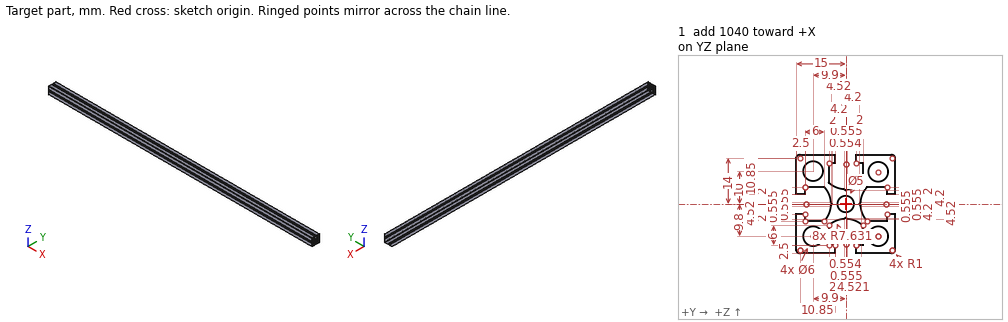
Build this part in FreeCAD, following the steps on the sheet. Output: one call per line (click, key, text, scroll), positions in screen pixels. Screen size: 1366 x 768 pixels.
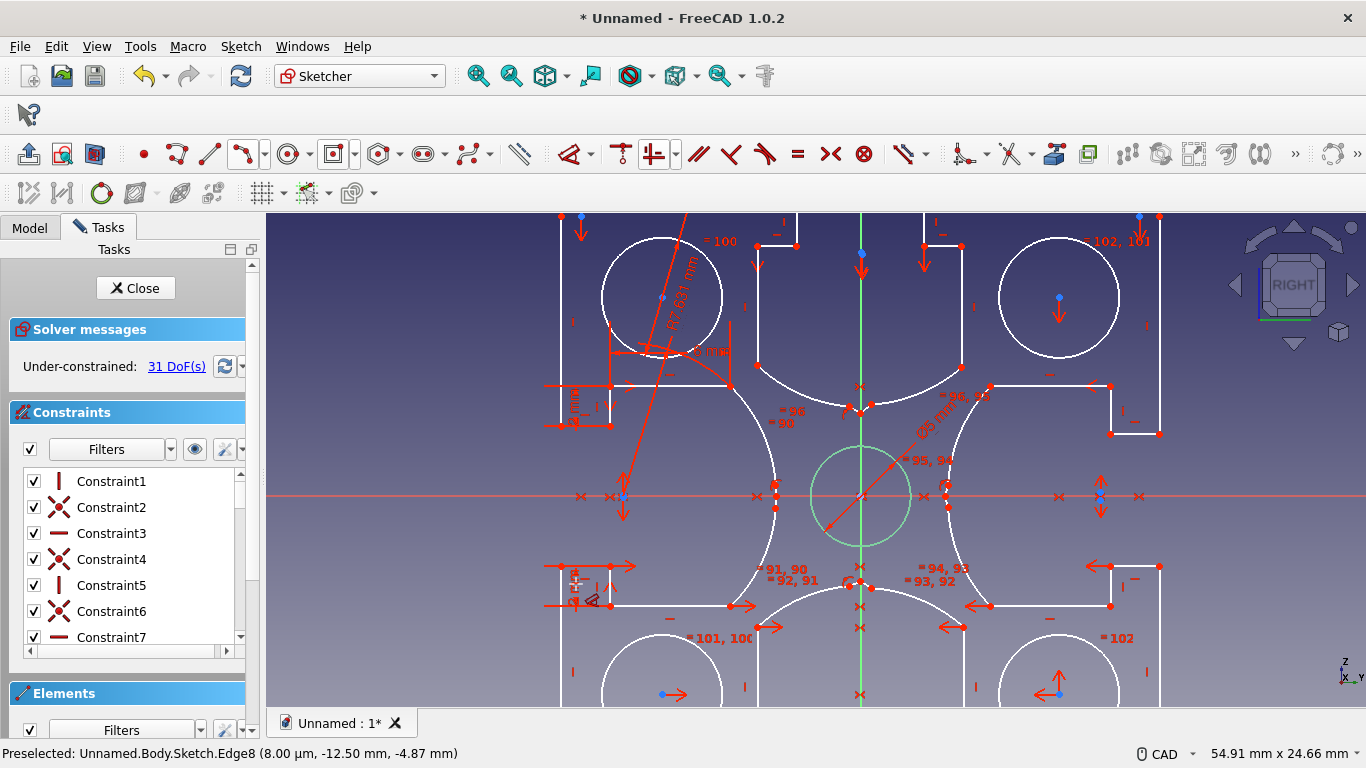
scroll(610, 416, down, 3)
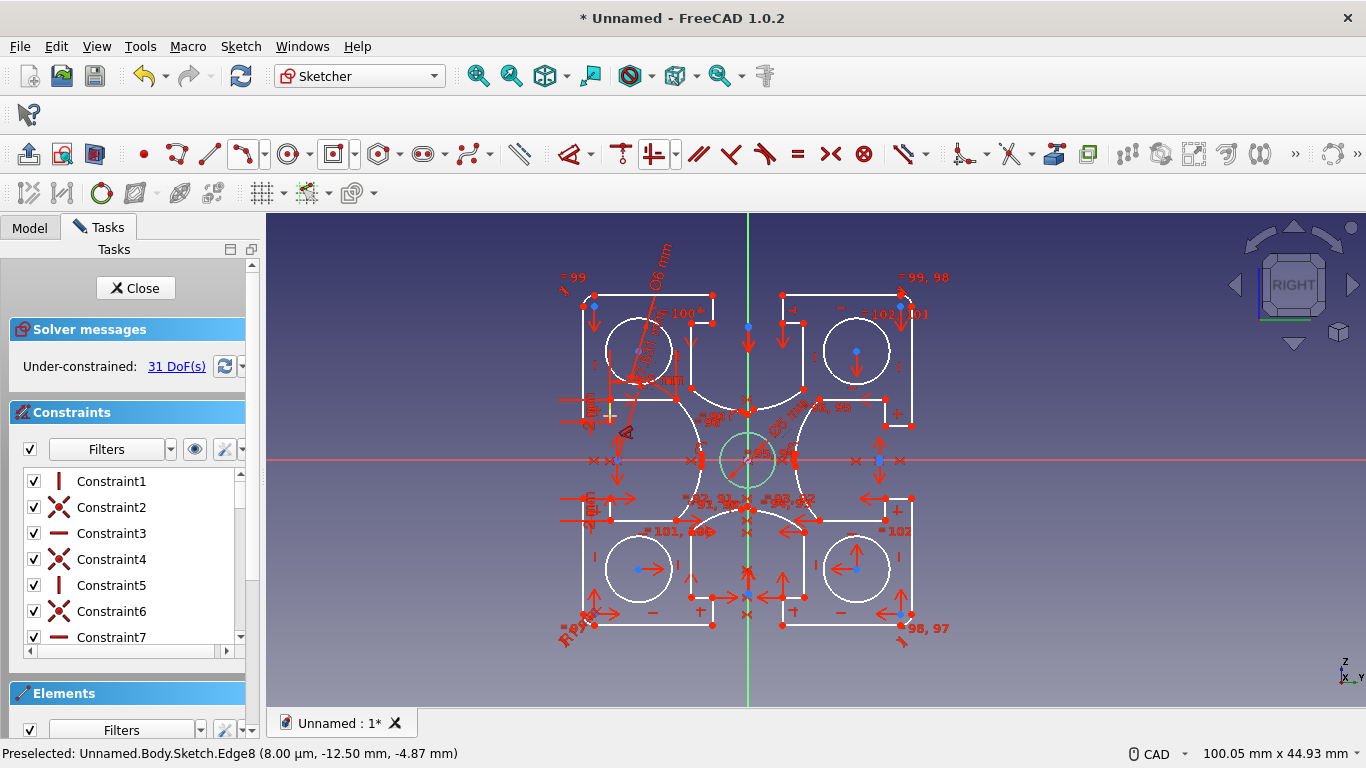
scroll(706, 598, up, 4)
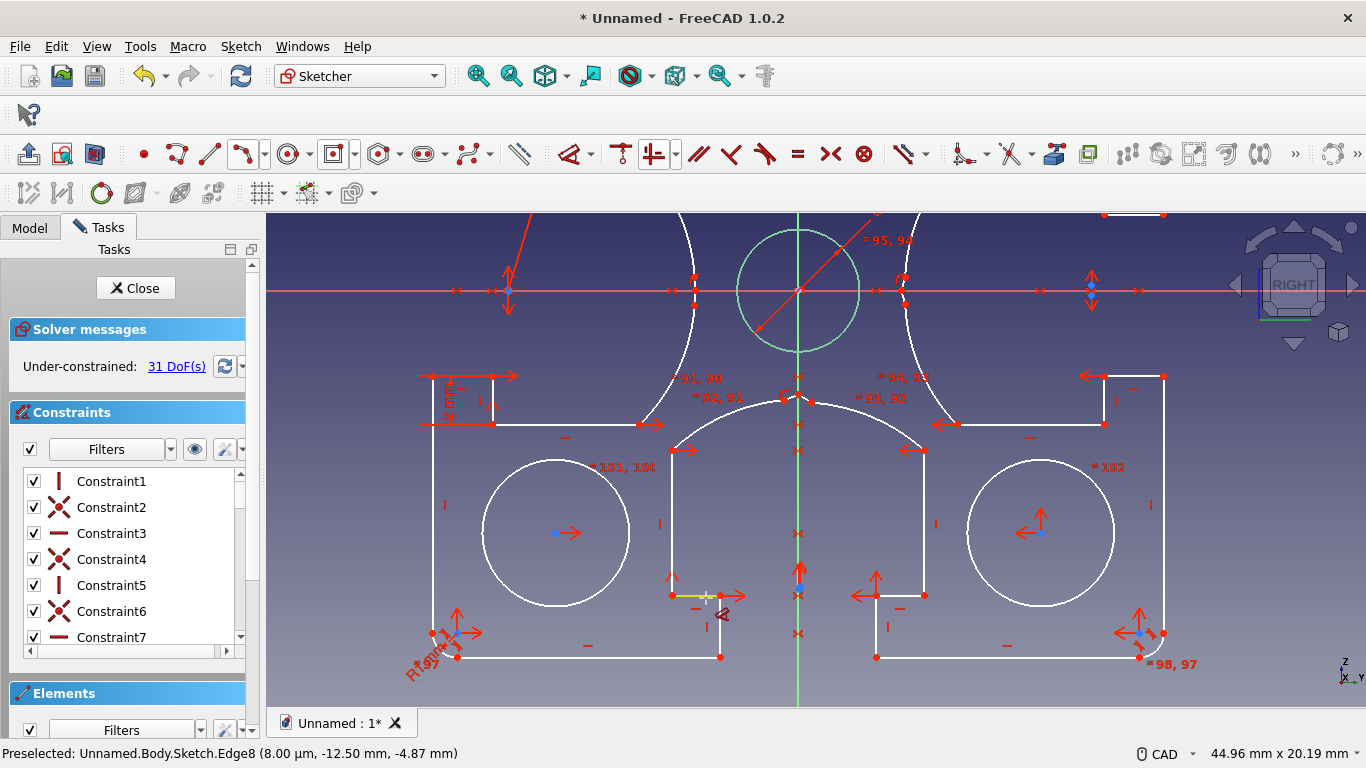
click(706, 596)
click(696, 630)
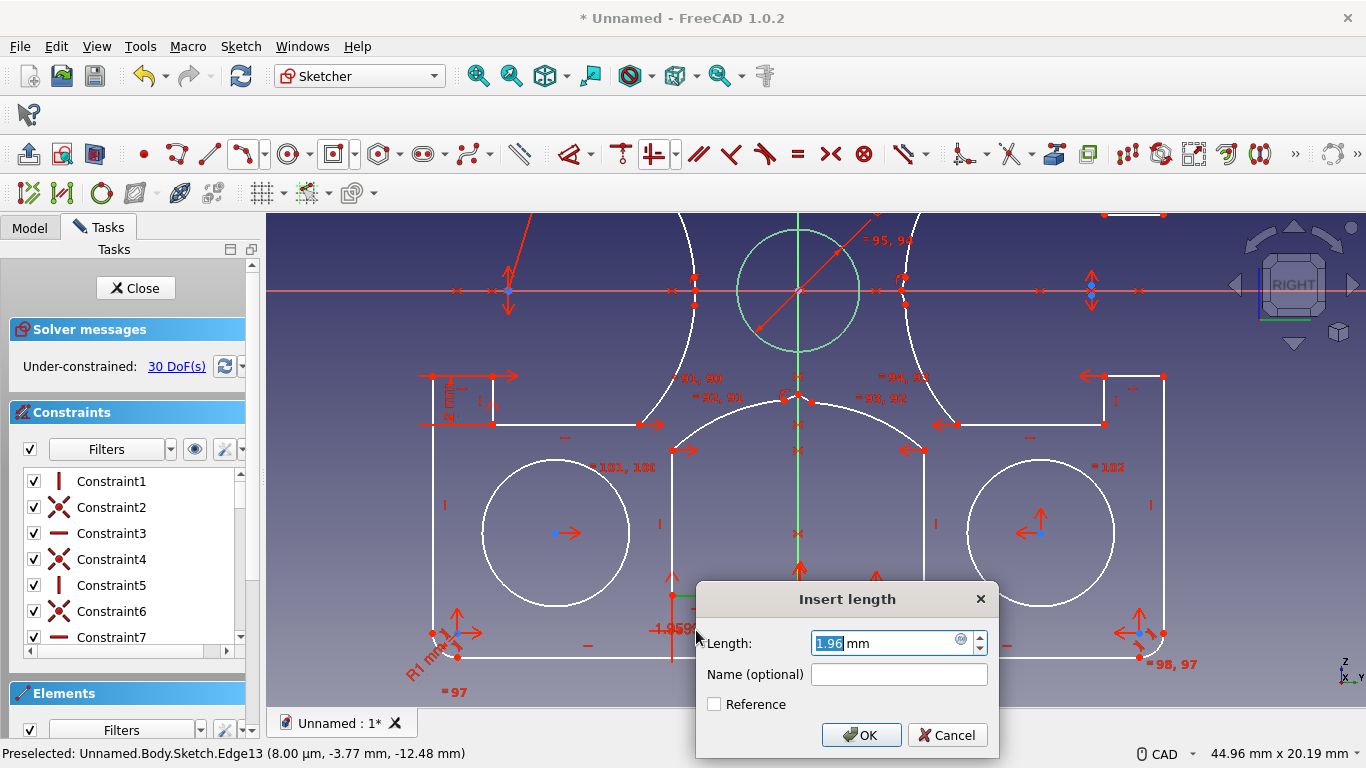
text(2)
key(Return)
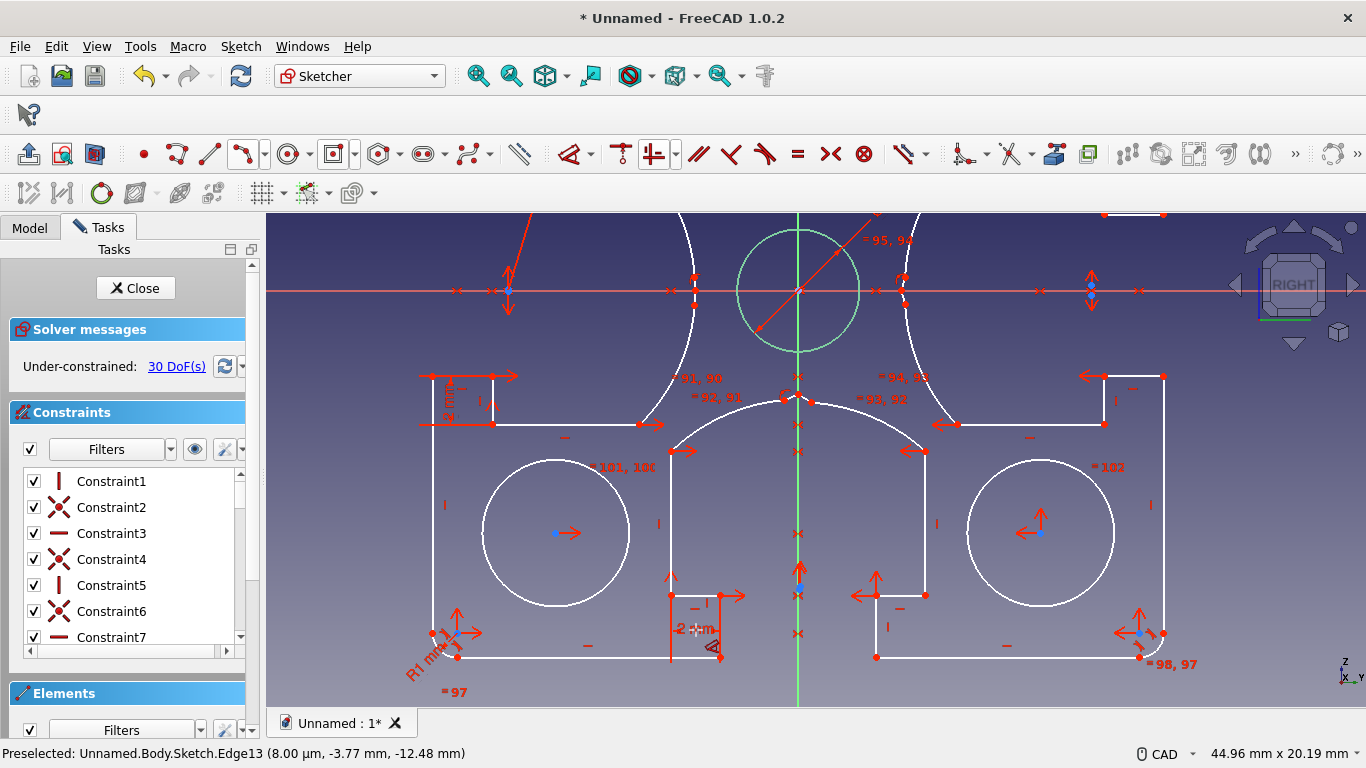
click(671, 553)
click(637, 490)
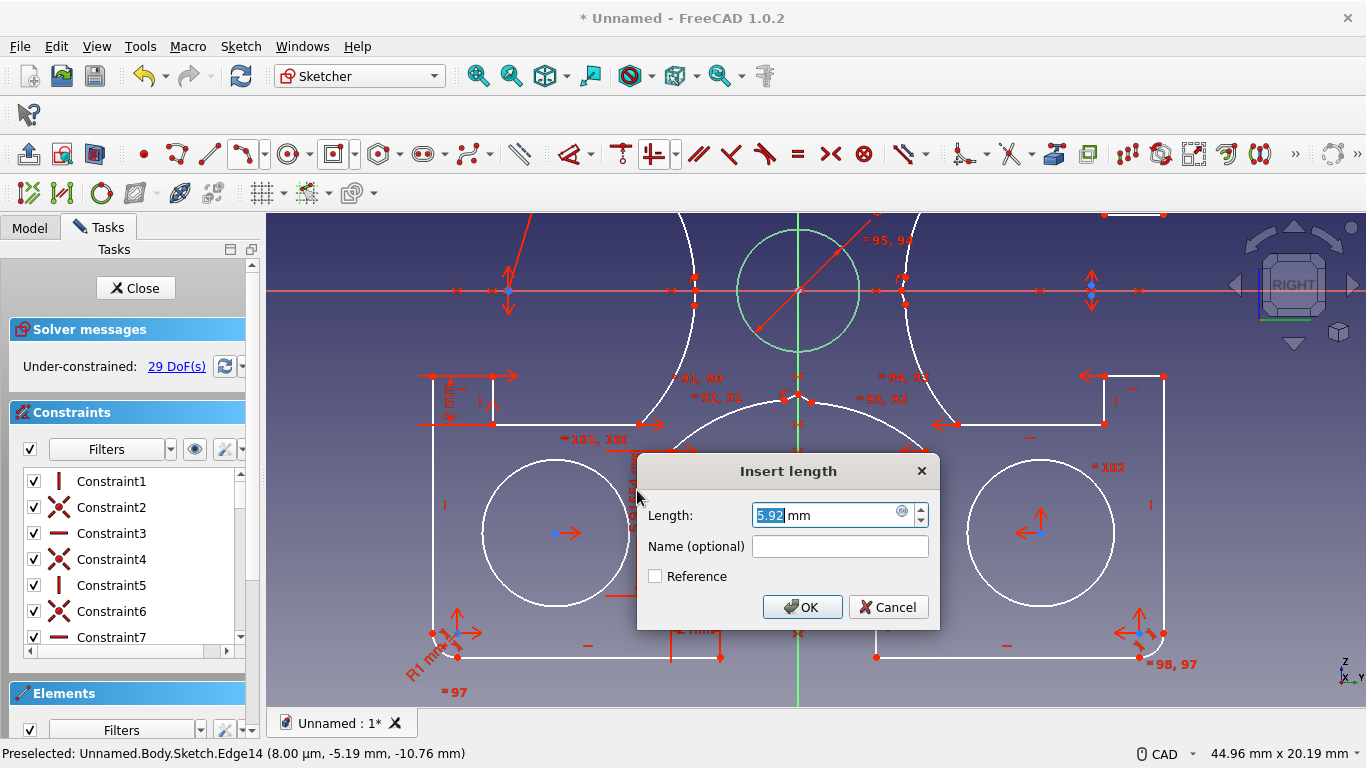
text(6)
key(Return)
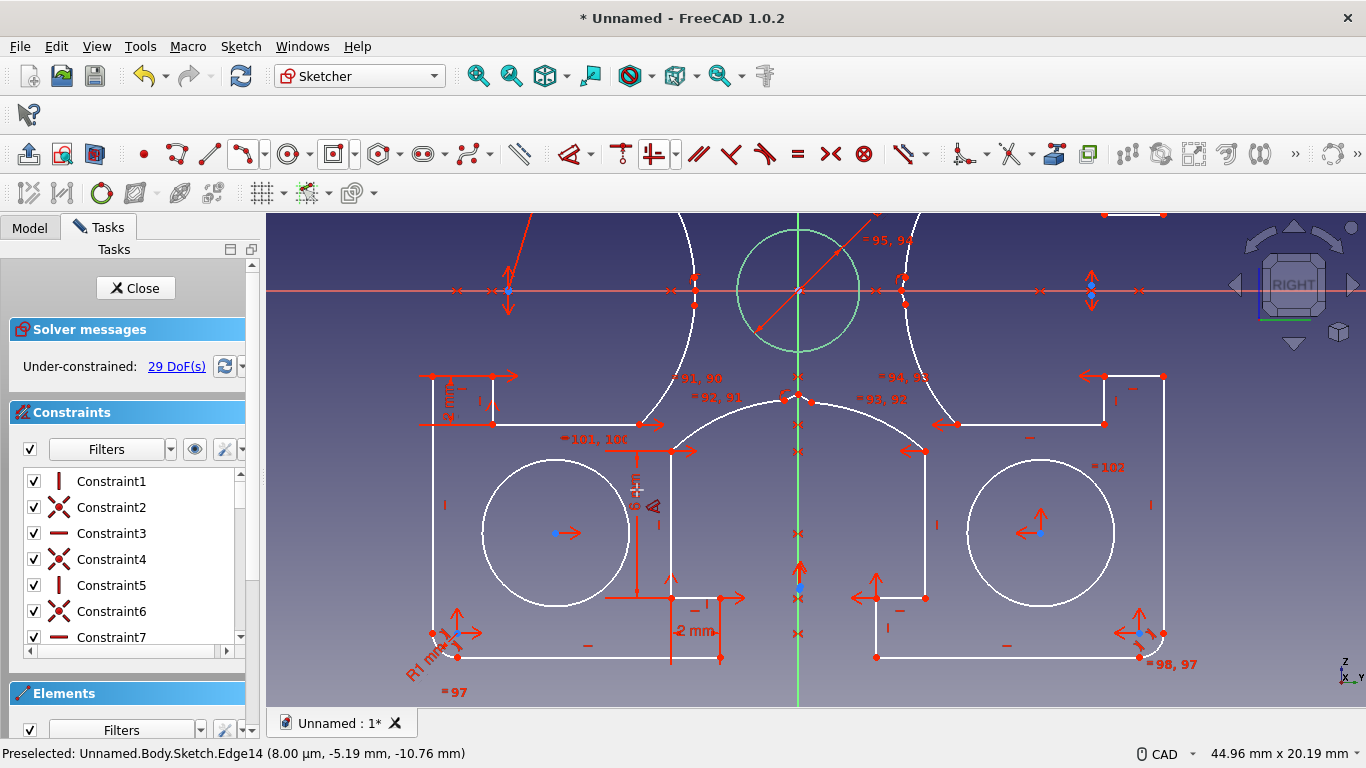
scroll(706, 598, down, 4)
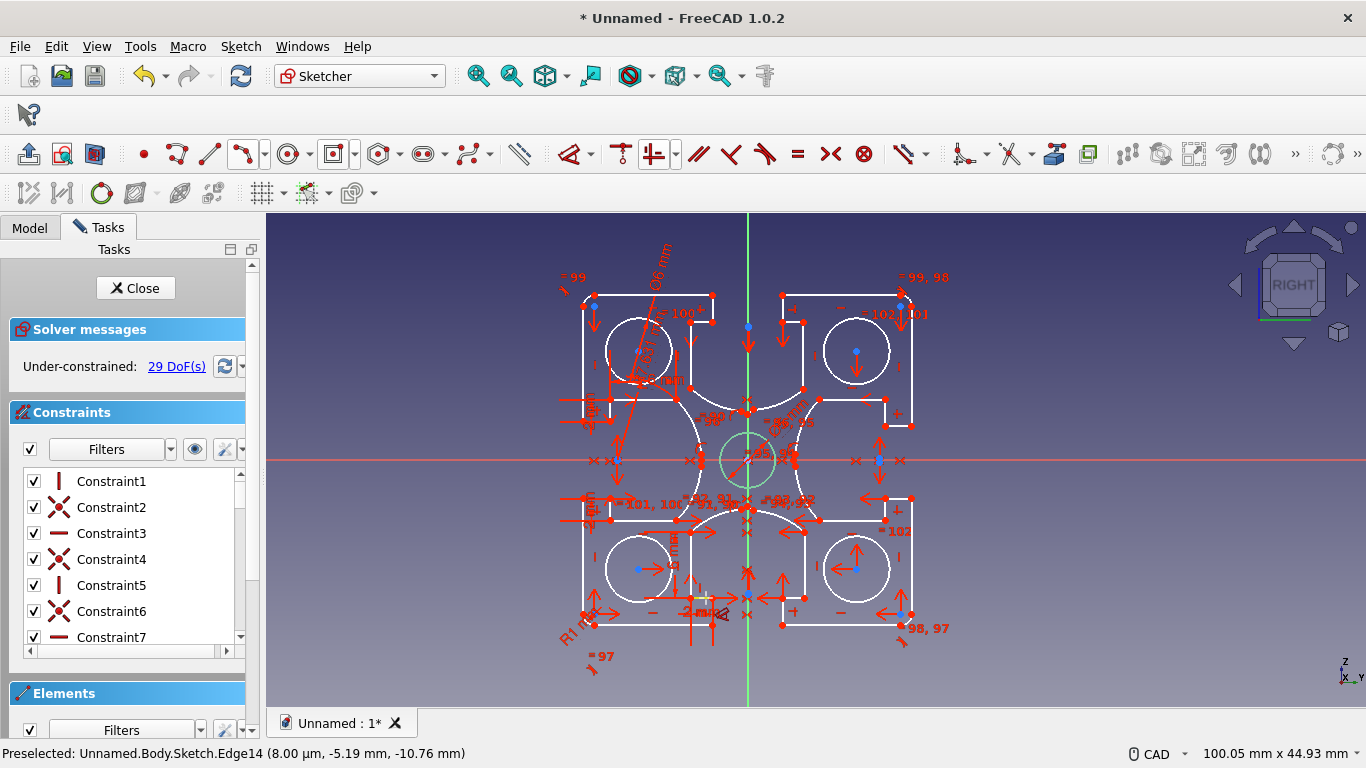
scroll(885, 408, up, 3)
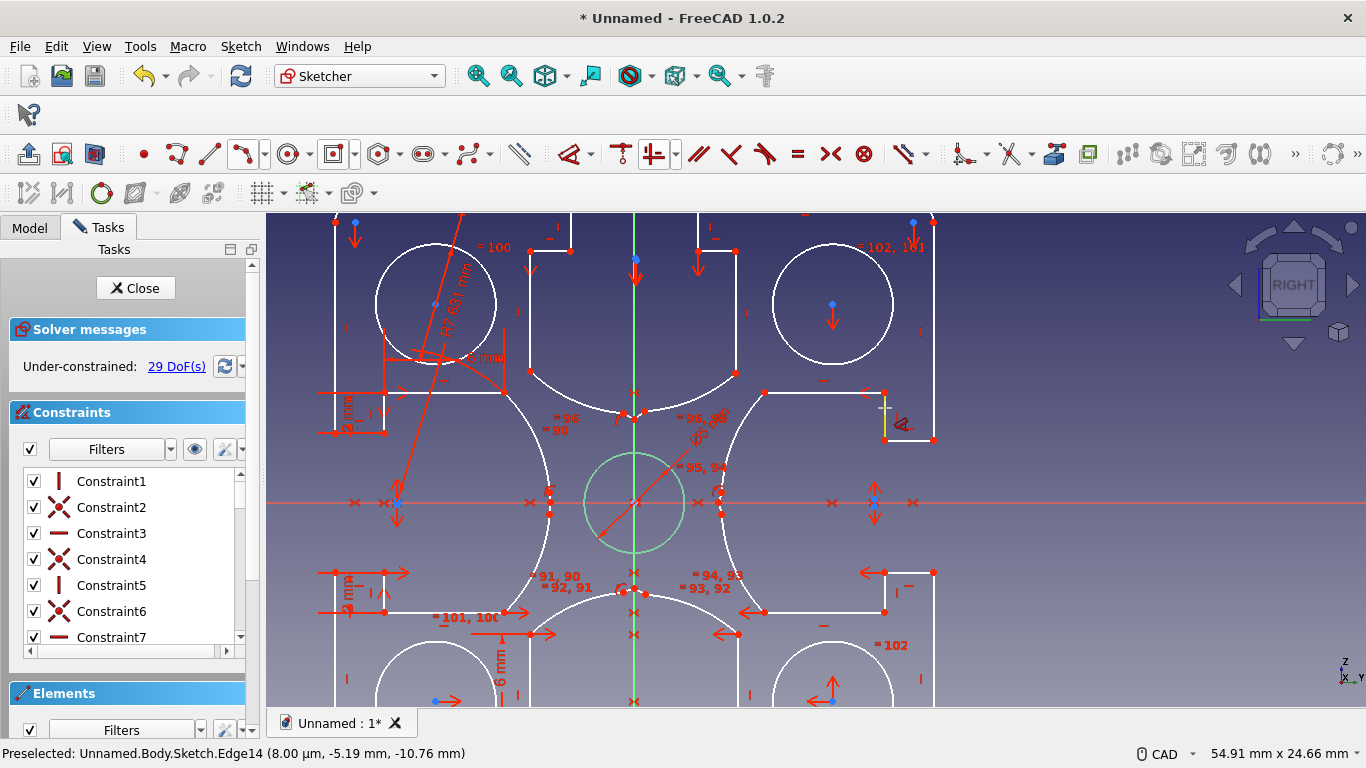
click(885, 407)
click(919, 417)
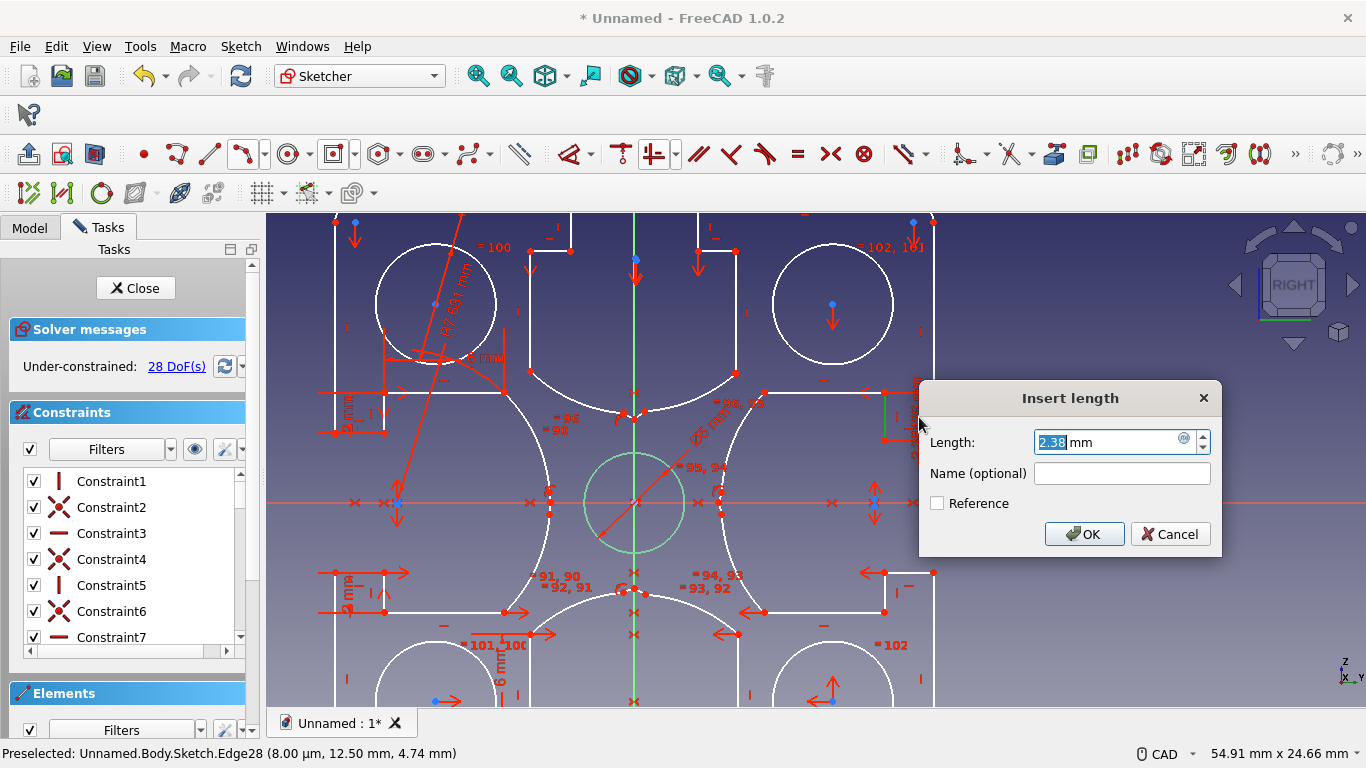
text(2)
key(Return)